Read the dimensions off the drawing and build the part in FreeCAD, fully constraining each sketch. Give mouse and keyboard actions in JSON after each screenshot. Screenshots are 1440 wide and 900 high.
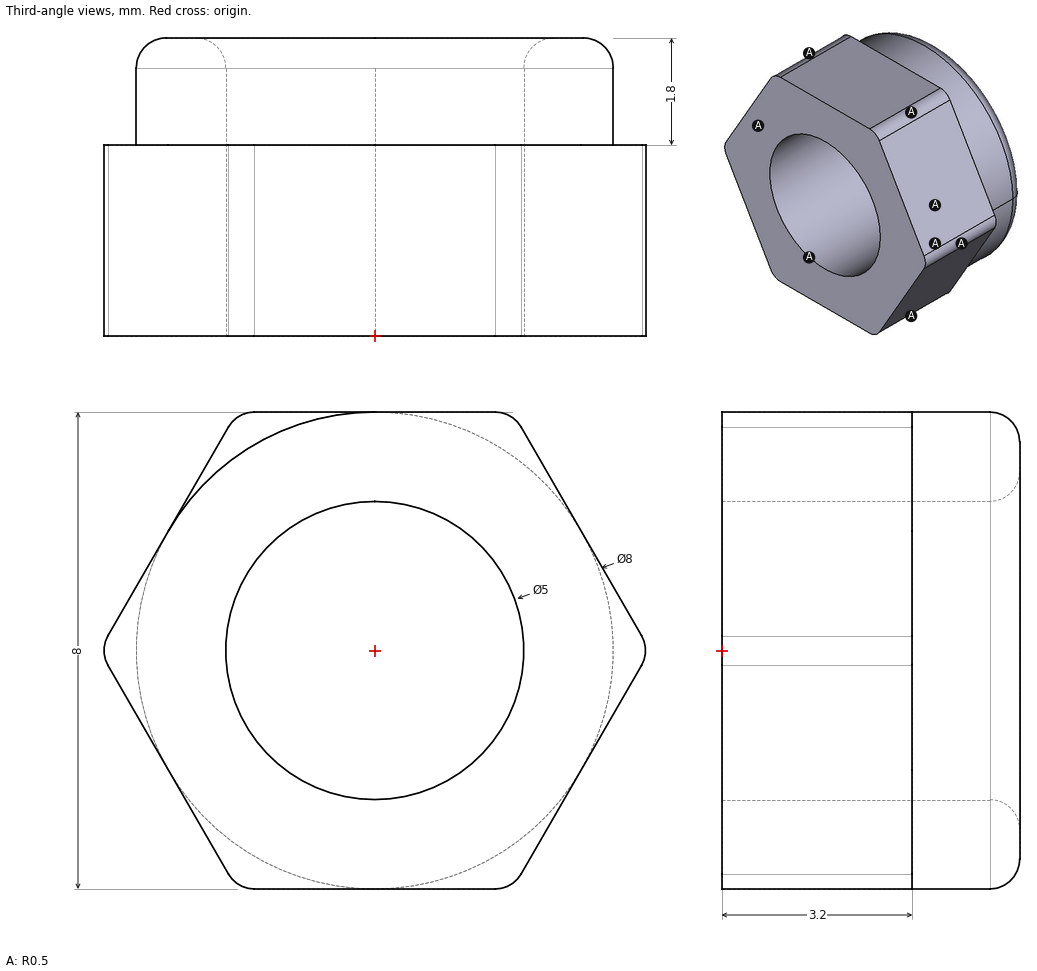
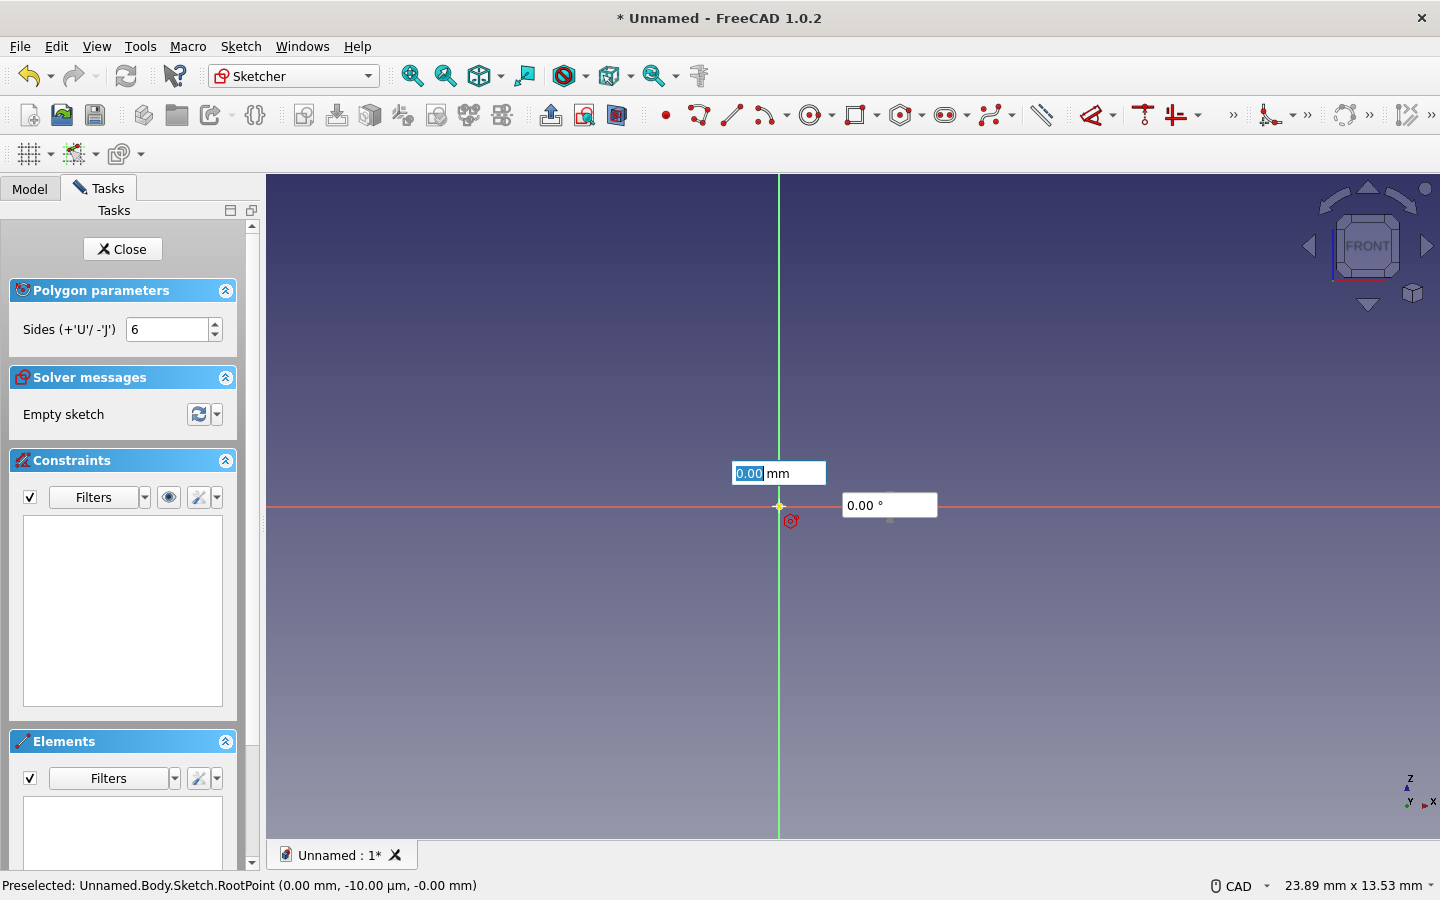
{"action": "left_click", "coordinate": [1006, 506]}
{"action": "right_click", "coordinate": [1006, 506]}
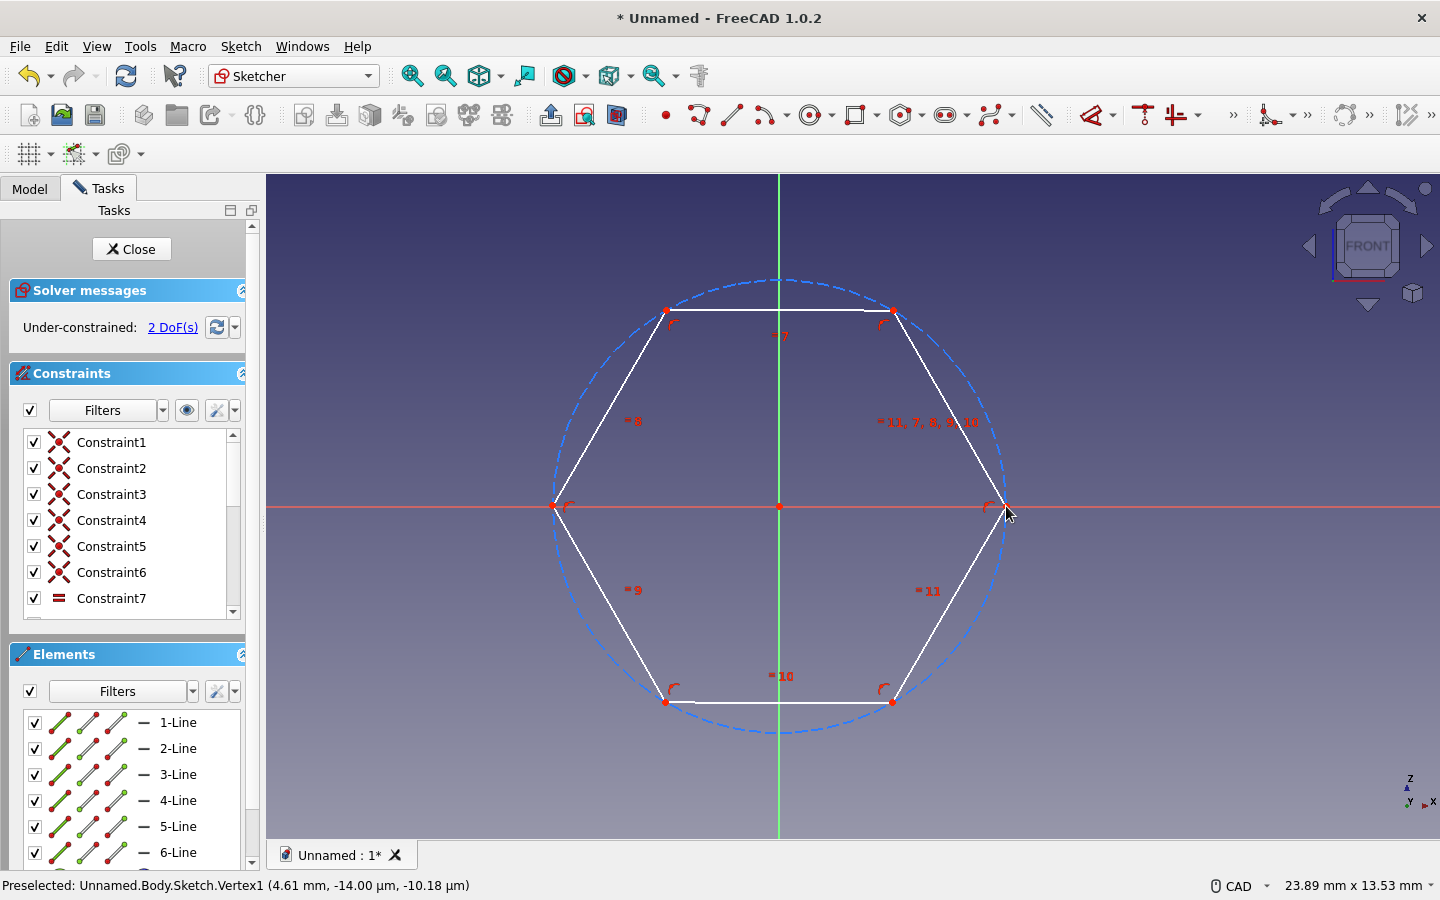
{"action": "left_click", "coordinate": [810, 116]}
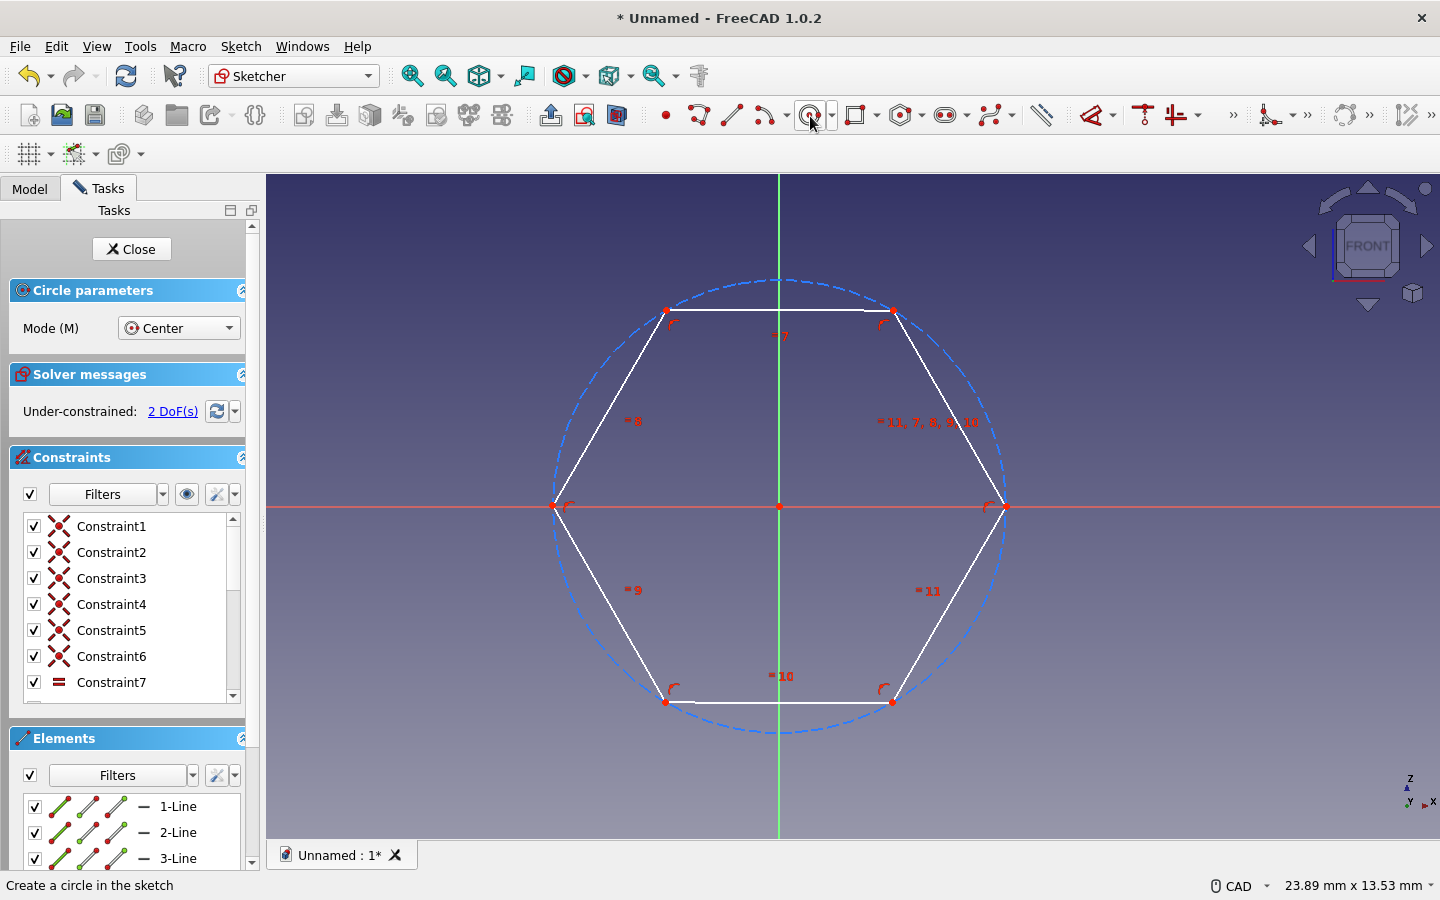
{"action": "left_click", "coordinate": [779, 506]}
{"action": "left_click", "coordinate": [866, 420]}
{"action": "key", "text": "Escape"}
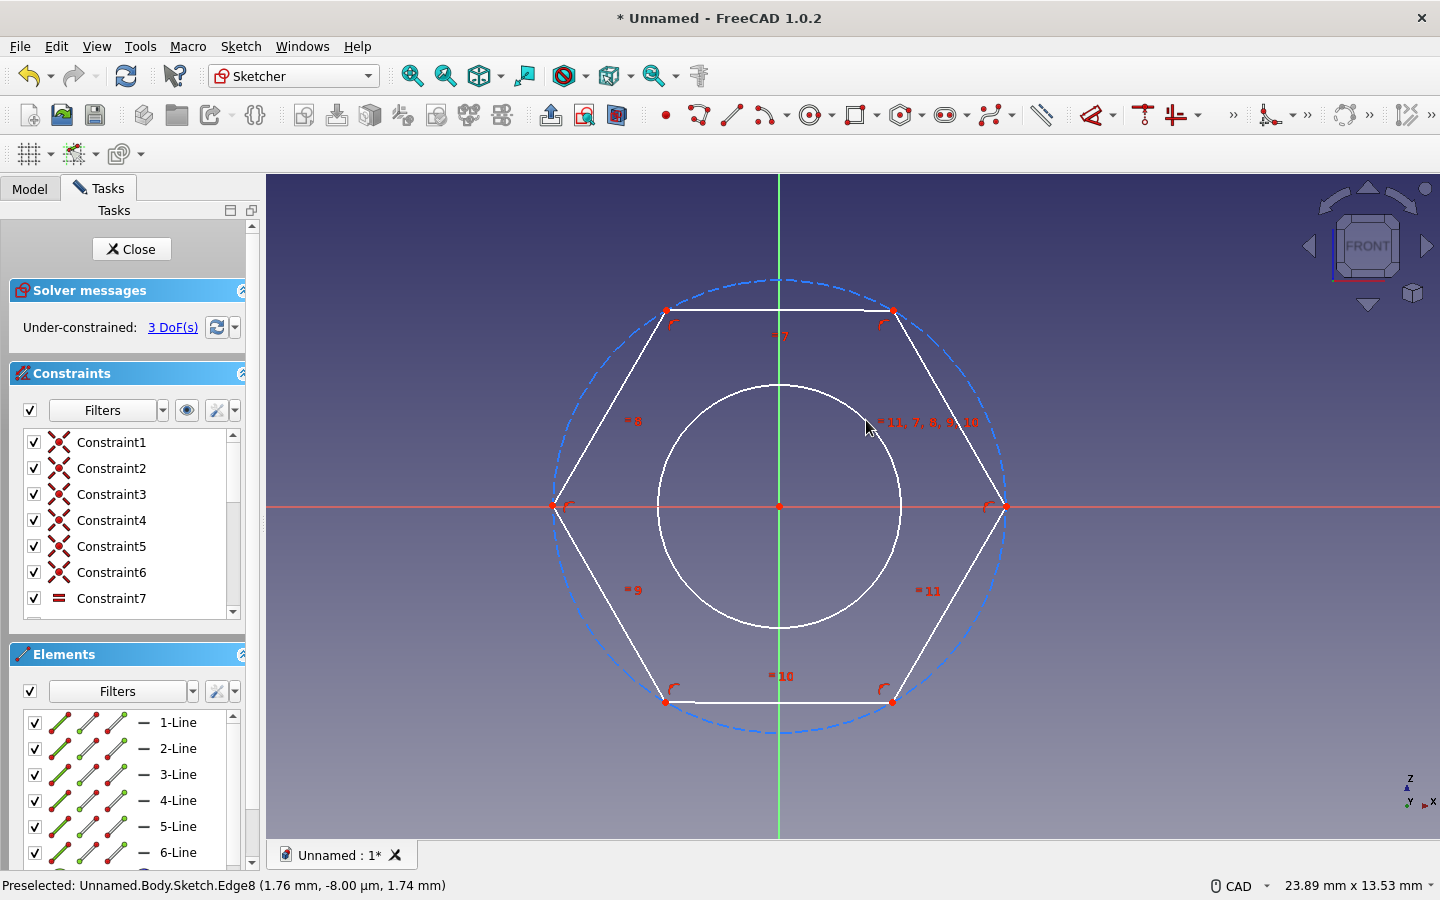
{"action": "left_click", "coordinate": [825, 310]}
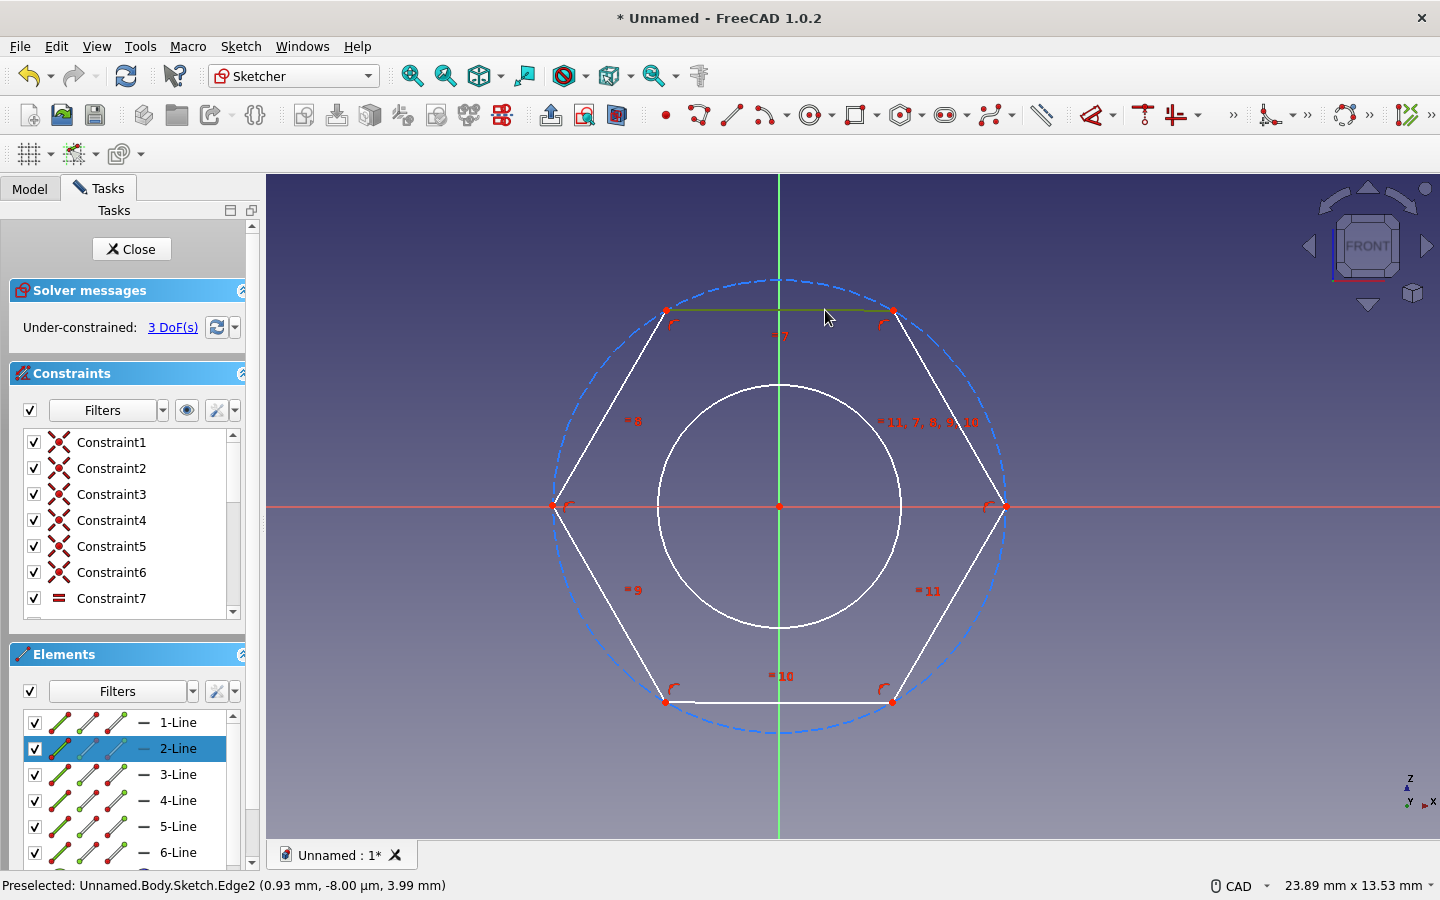
{"action": "key", "text": "h"}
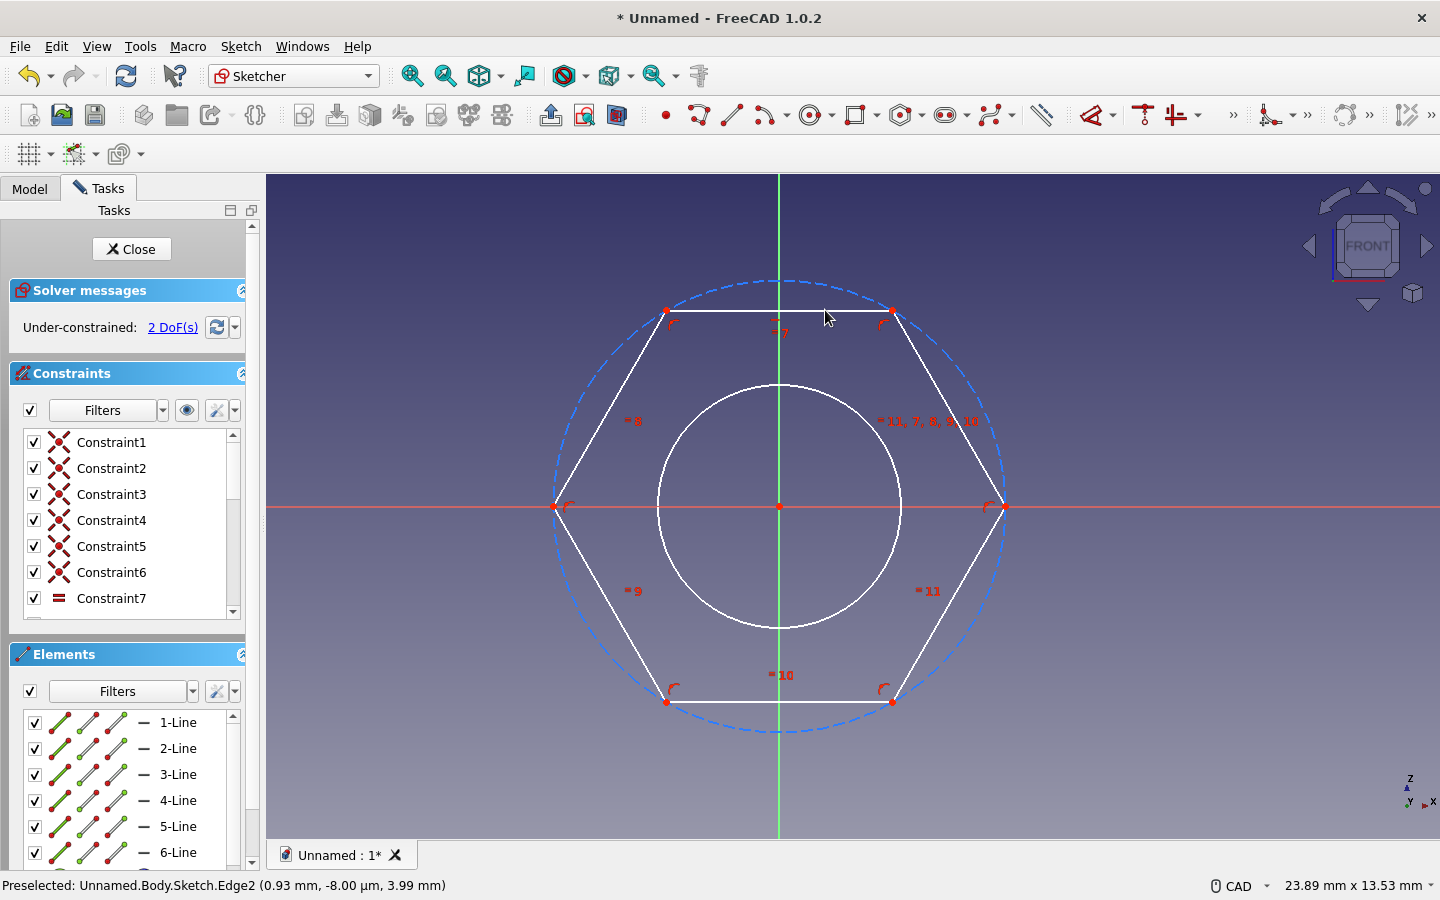
{"action": "left_click", "coordinate": [865, 420]}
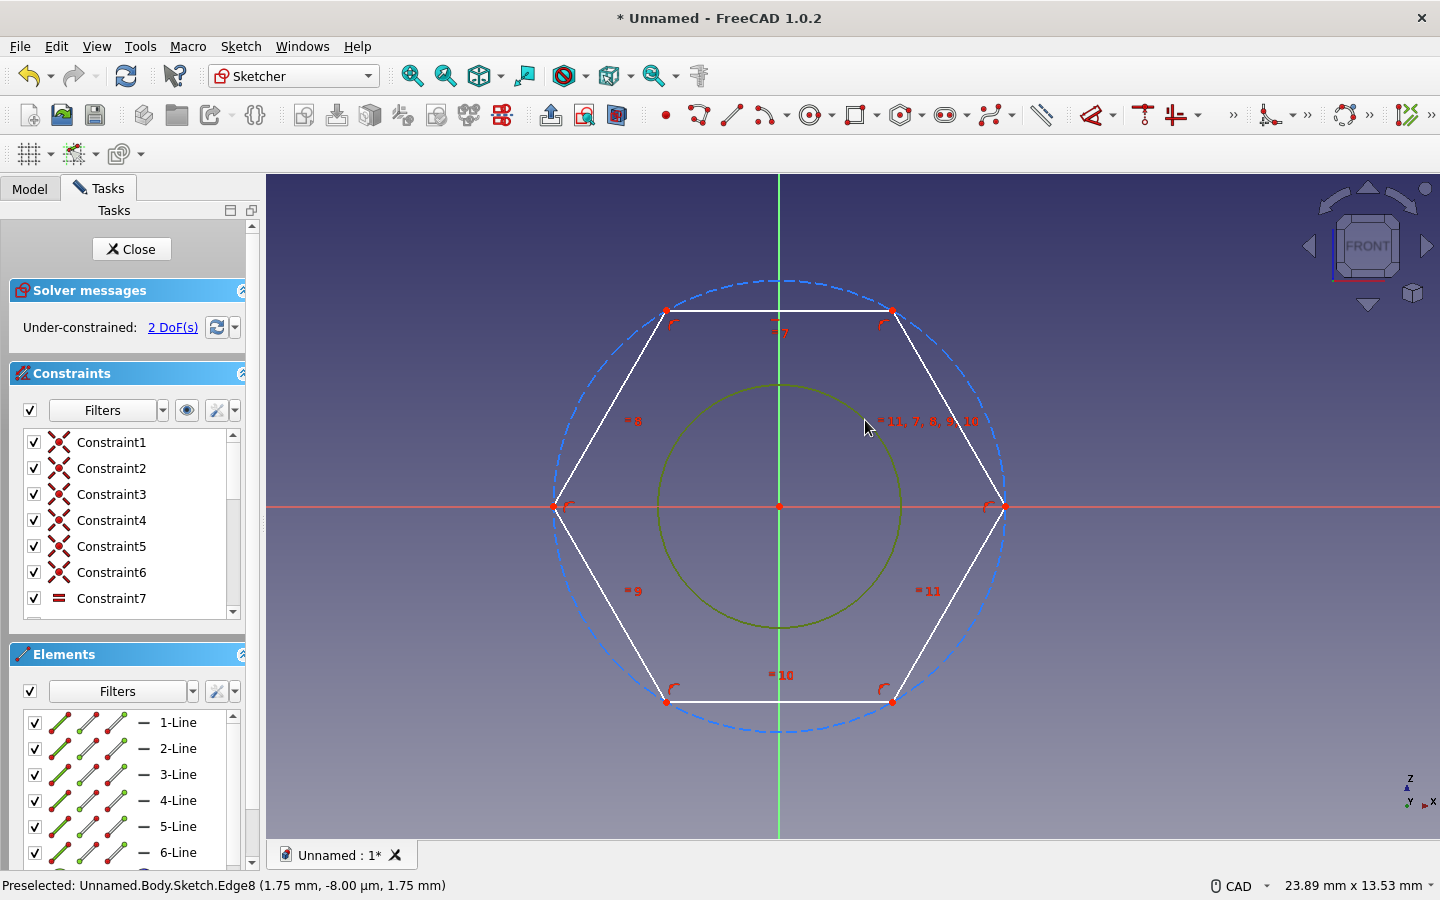
{"action": "left_click", "coordinate": [1112, 116]}